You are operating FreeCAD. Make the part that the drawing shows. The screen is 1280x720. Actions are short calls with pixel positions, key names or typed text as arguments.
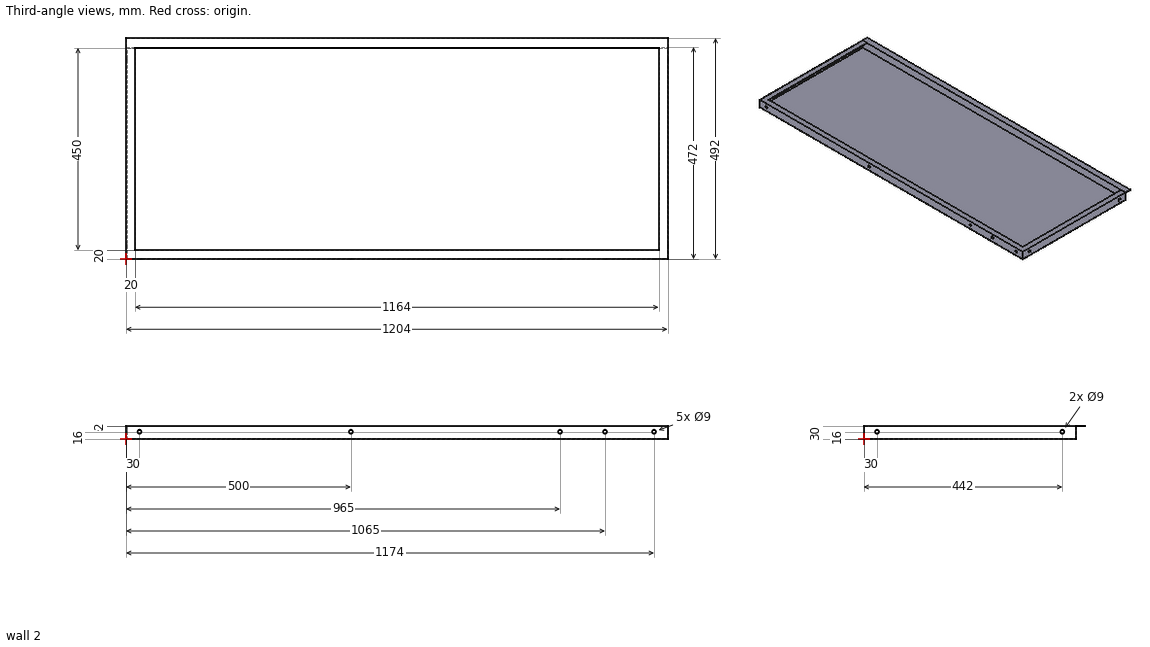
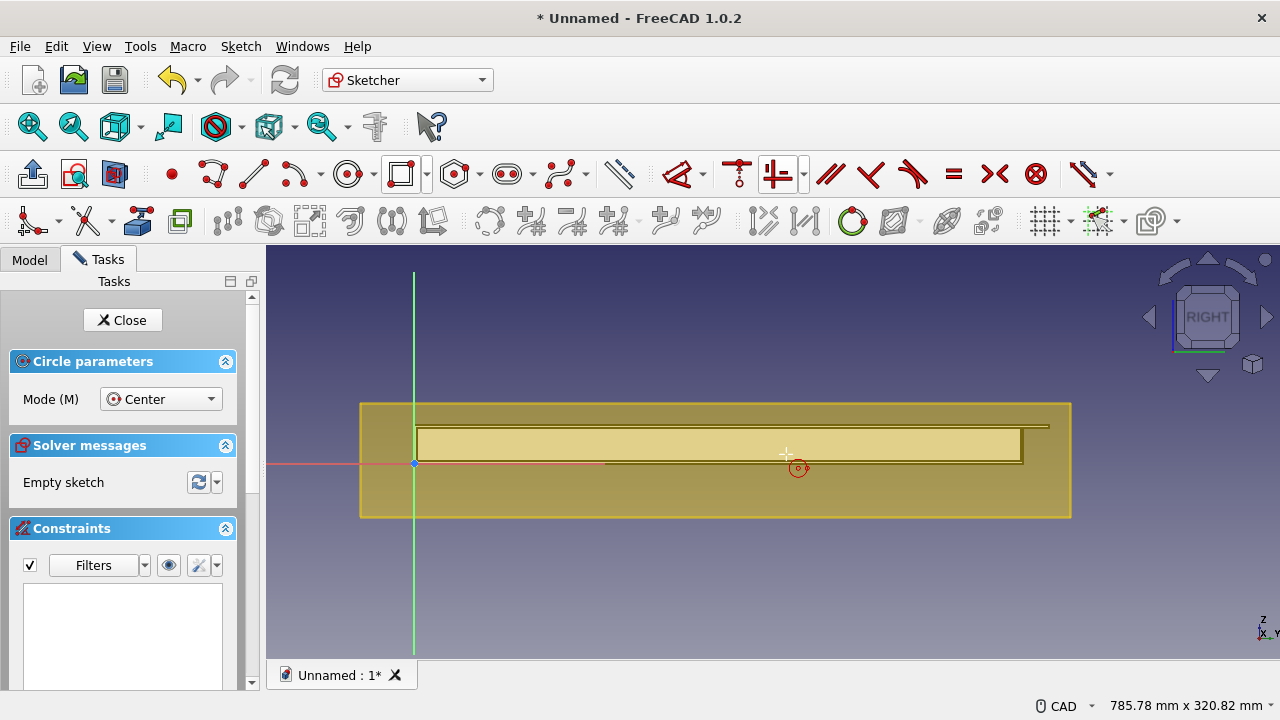
scroll(985, 443, up, 7)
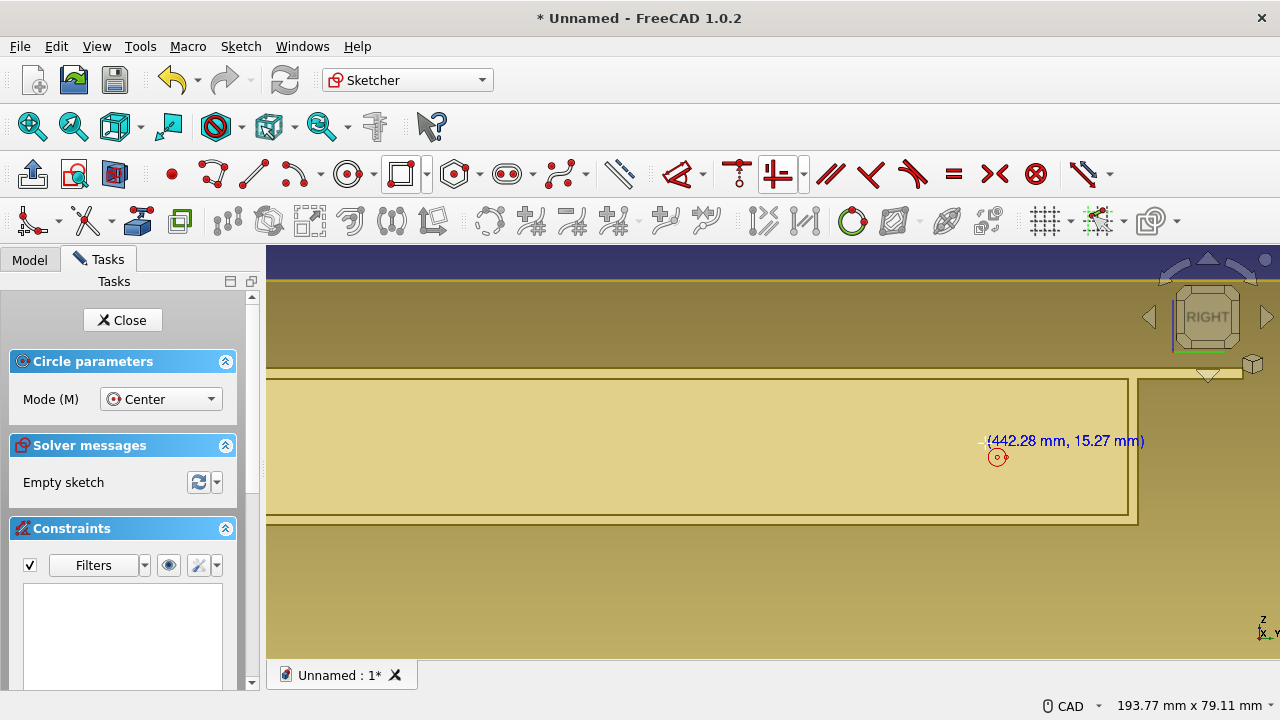
scroll(989, 446, down, 7)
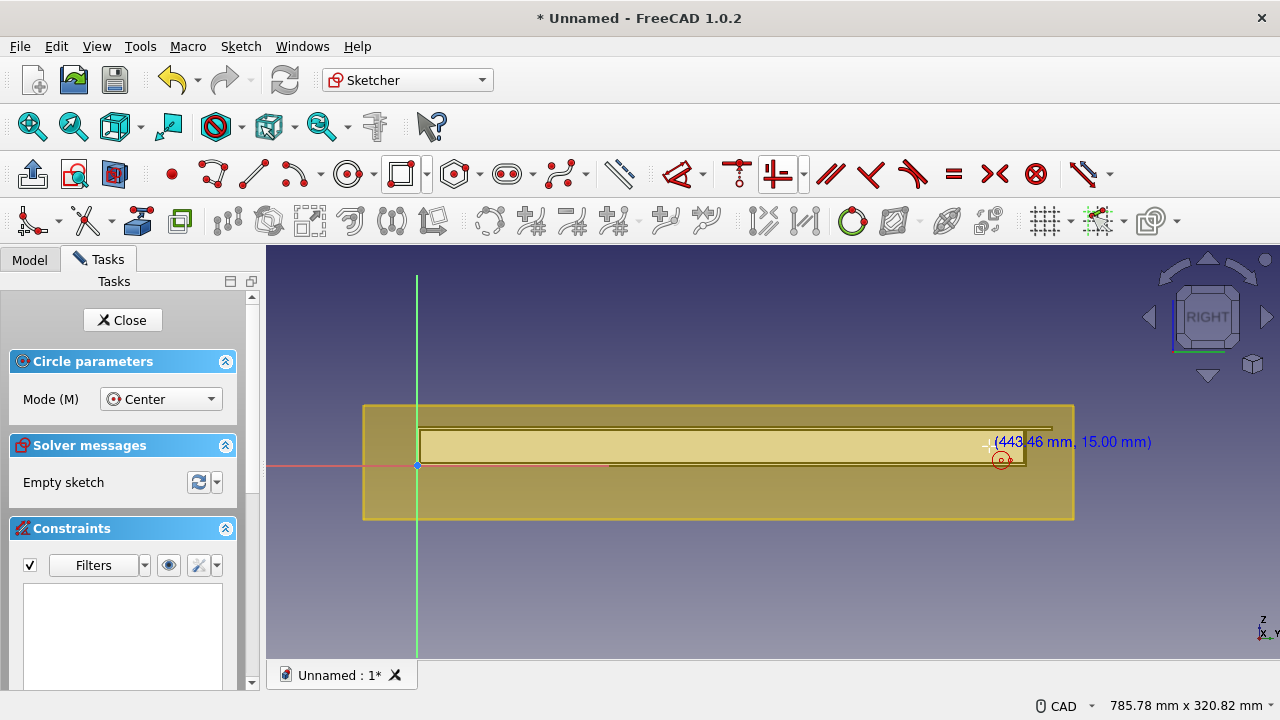
click(988, 445)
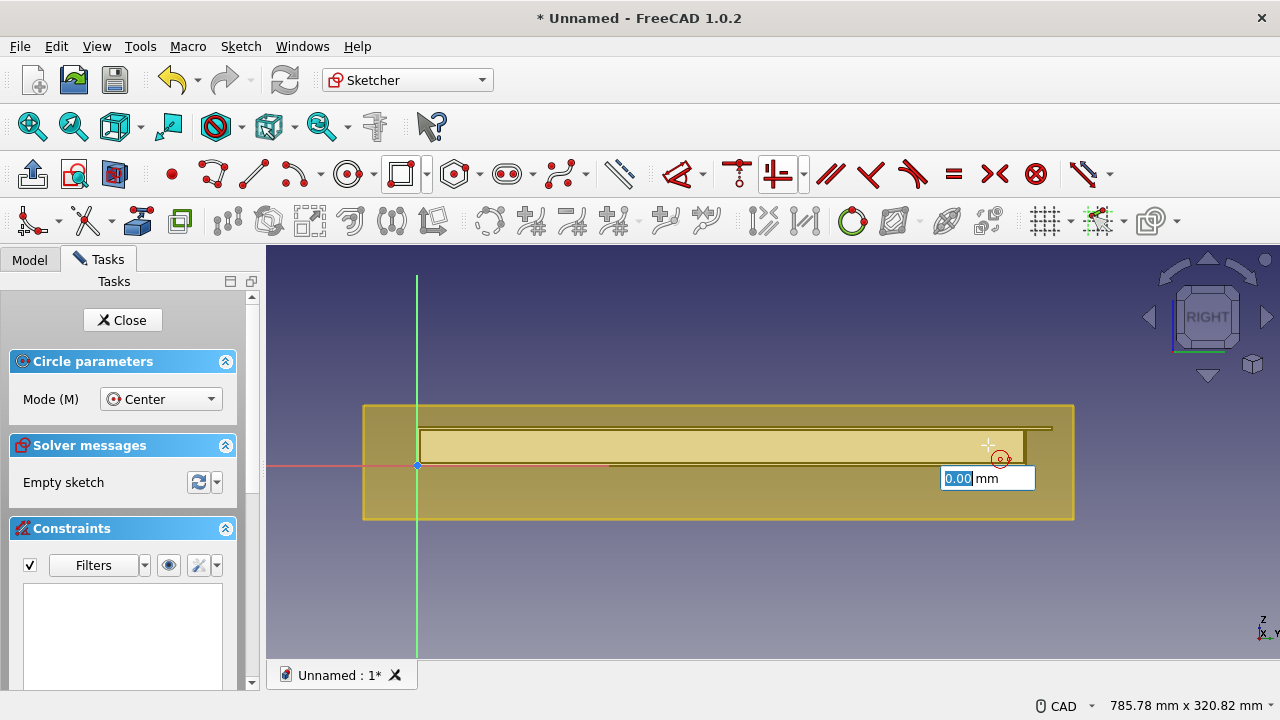
scroll(992, 441, up, 6)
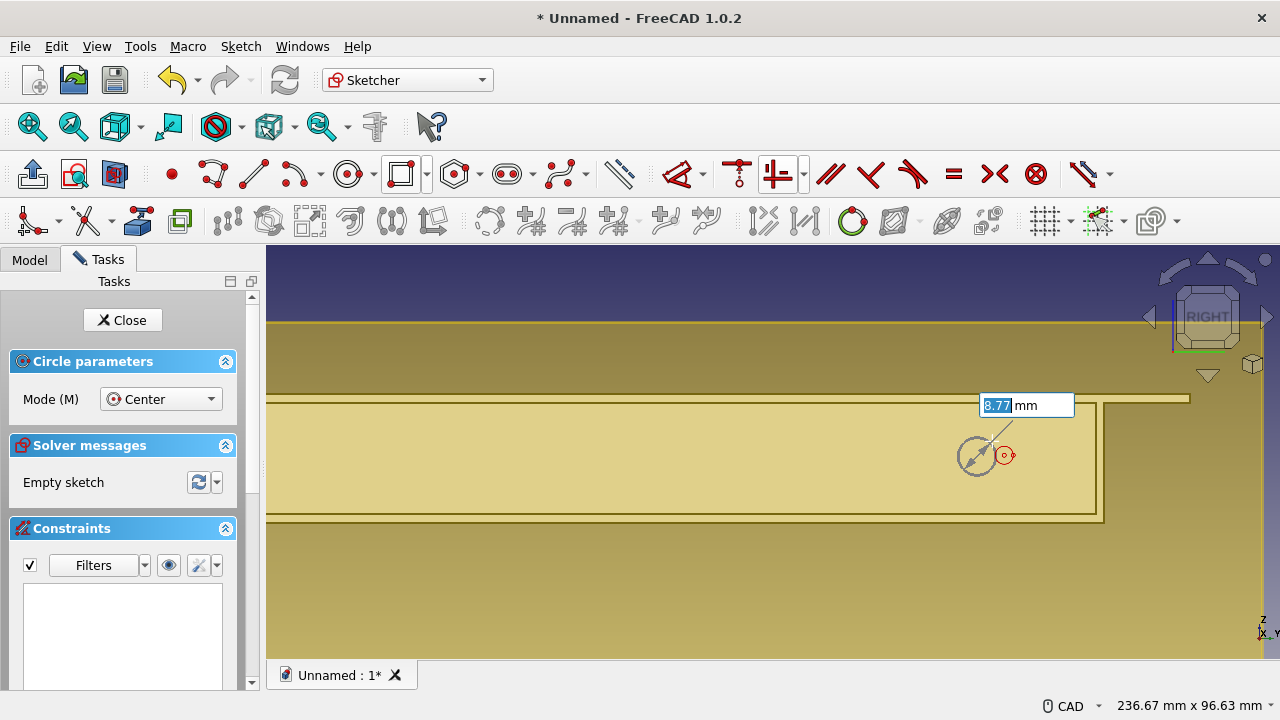
click(990, 441)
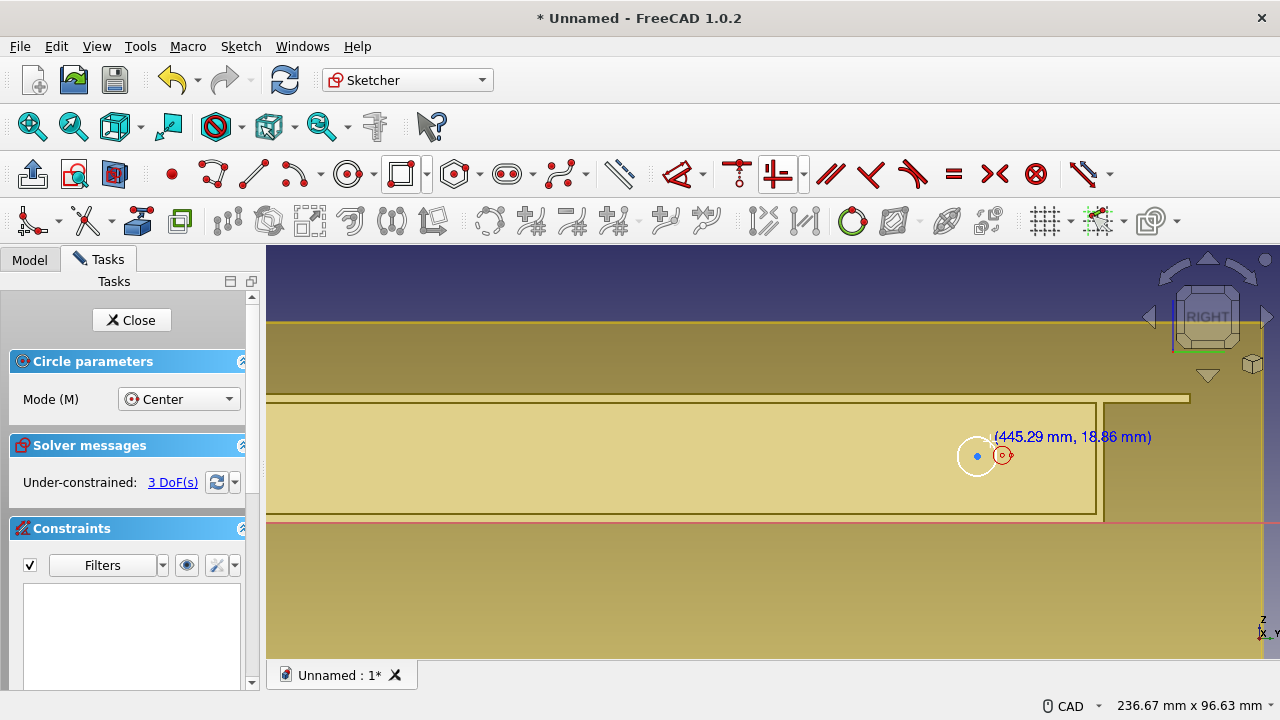
scroll(991, 440, down, 6)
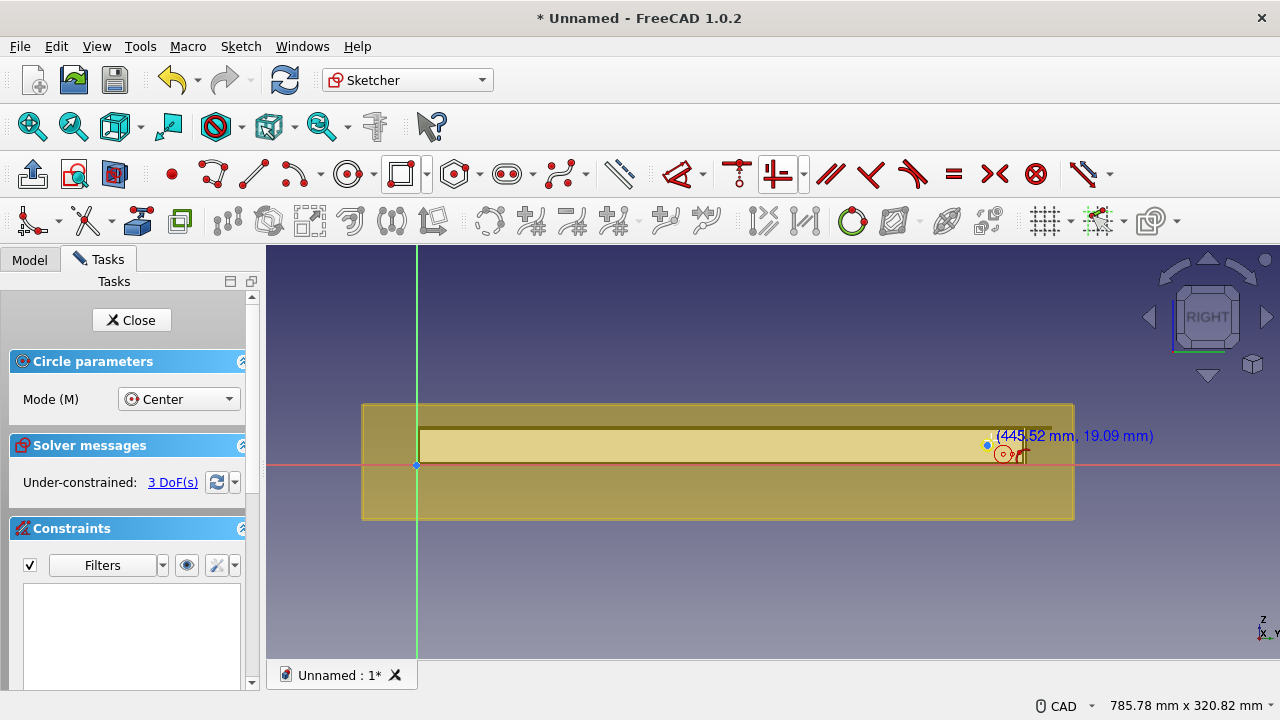
scroll(455, 445, up, 7)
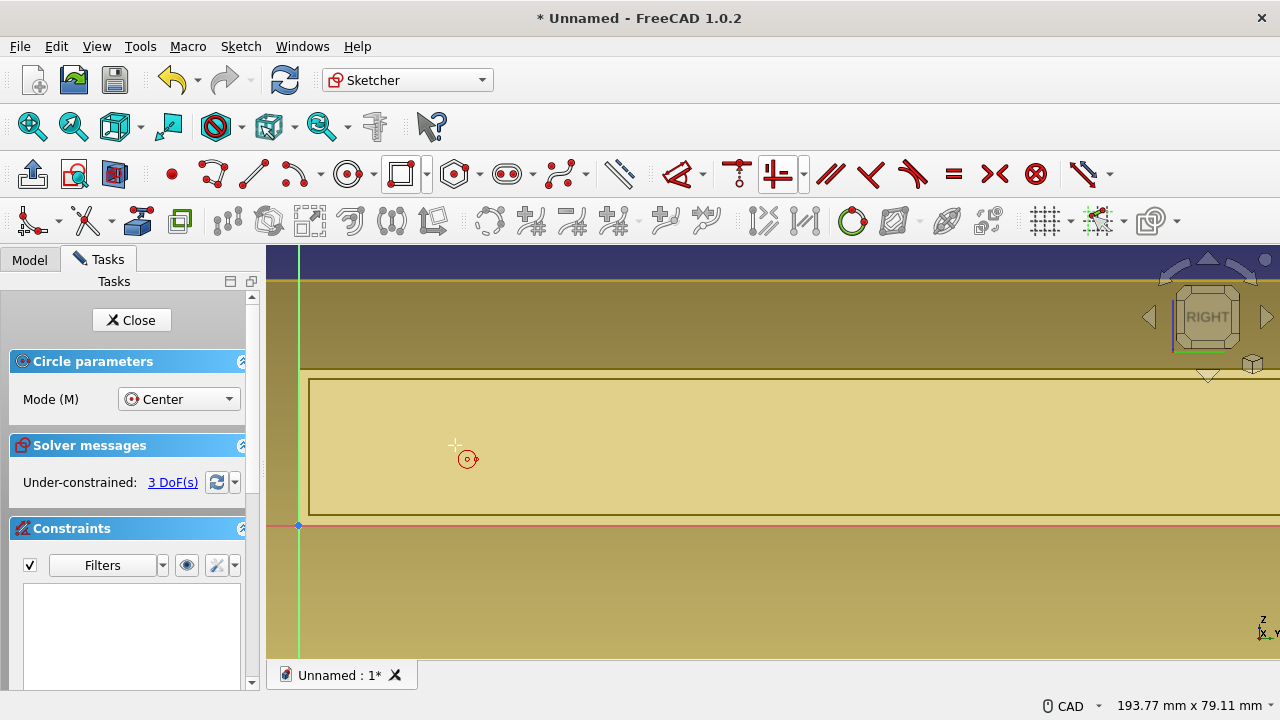
scroll(455, 445, down, 7)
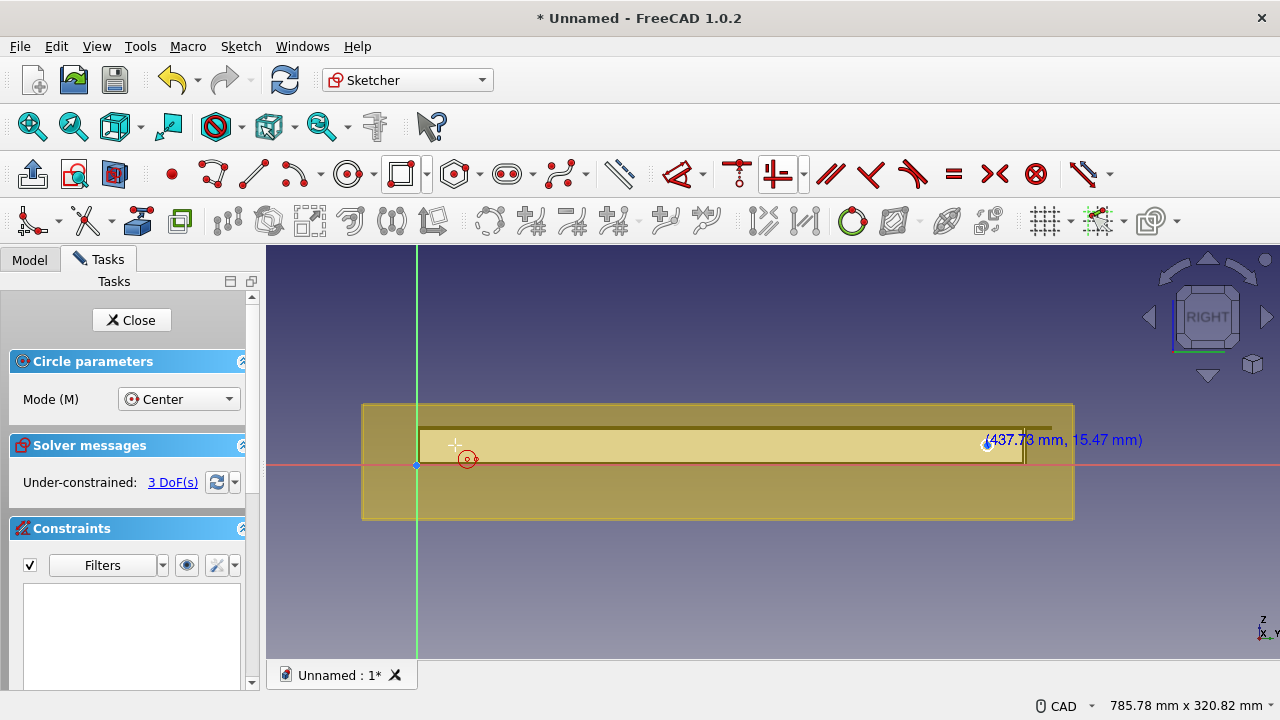
click(455, 445)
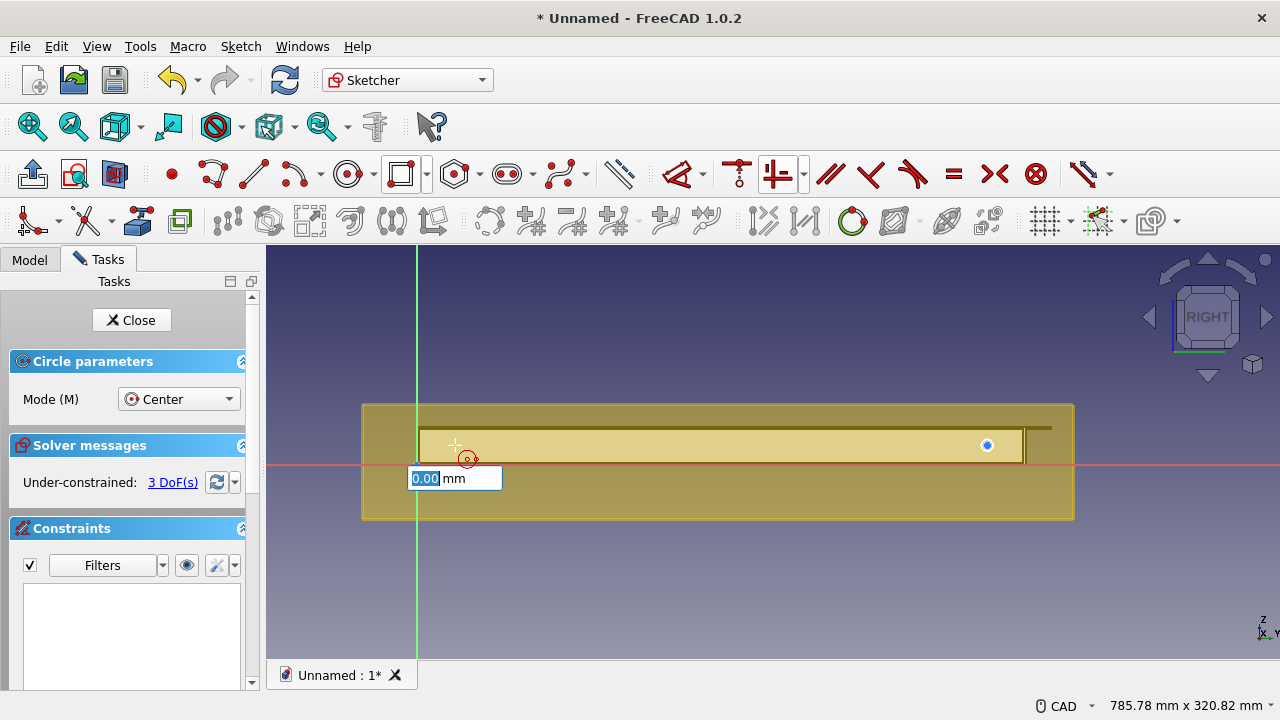
scroll(459, 441, up, 6)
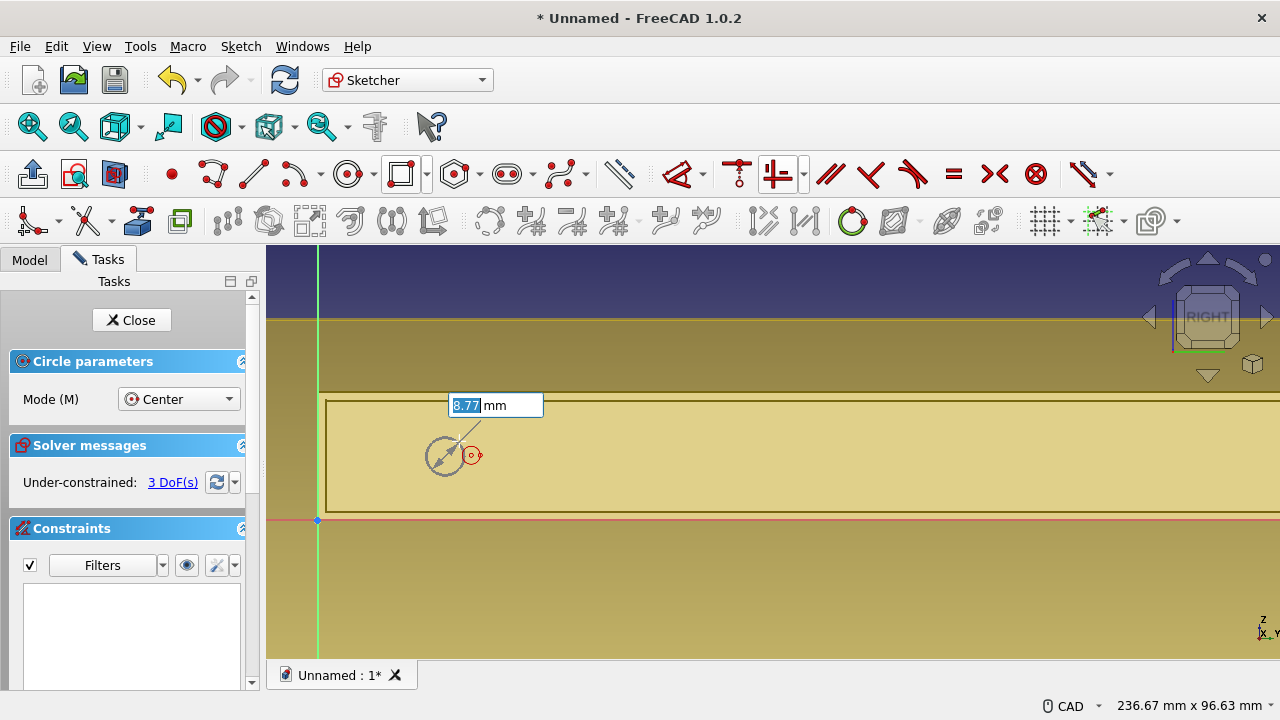
click(460, 438)
key(Escape)